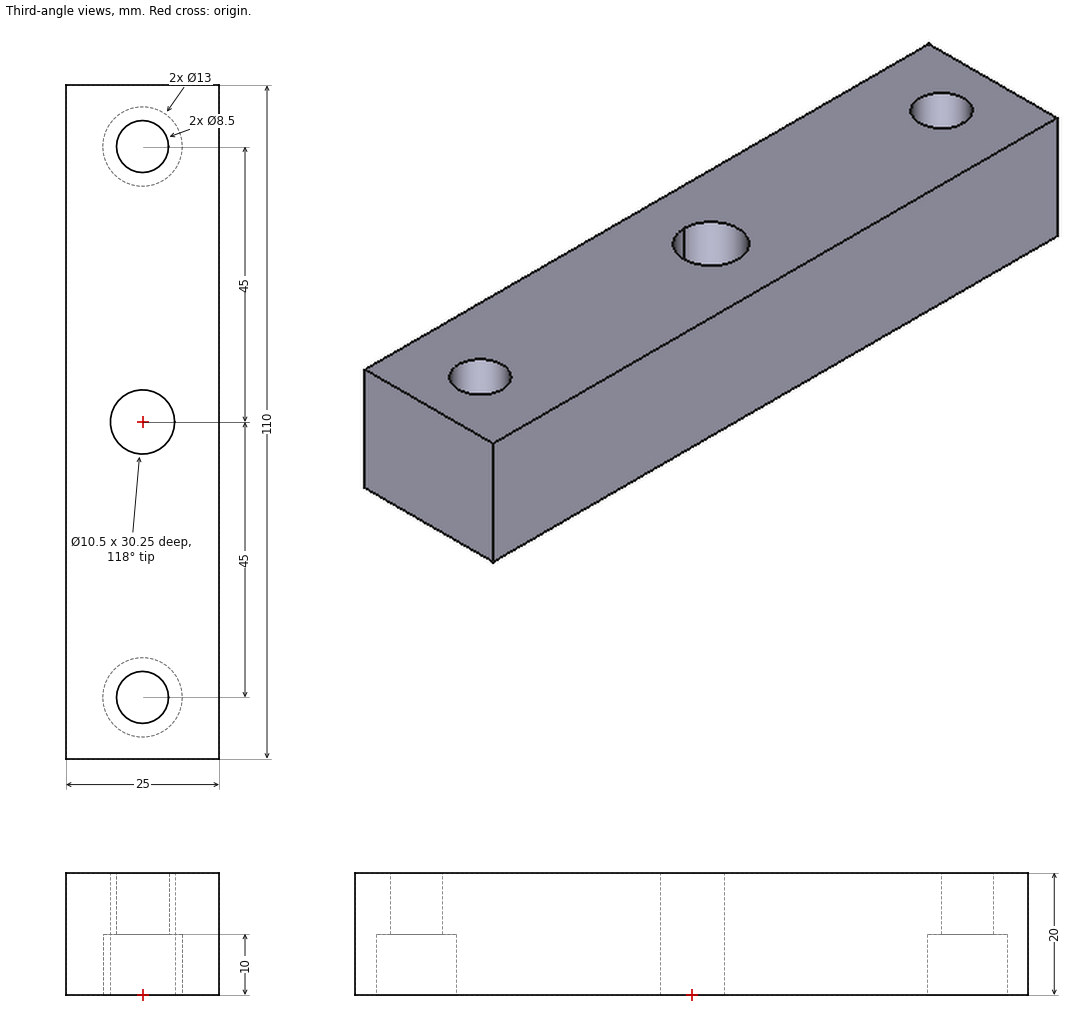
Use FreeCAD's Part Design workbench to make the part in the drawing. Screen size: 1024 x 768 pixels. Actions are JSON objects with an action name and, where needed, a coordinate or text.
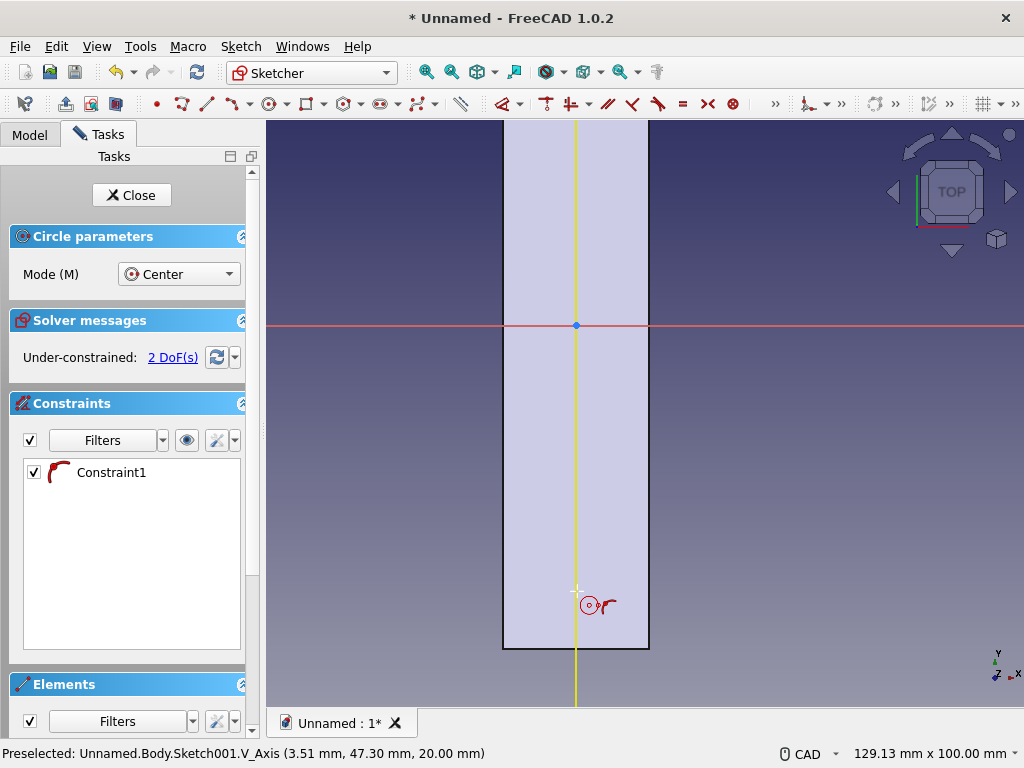
{"action": "left_click", "coordinate": [576, 590]}
{"action": "left_click", "coordinate": [594, 572]}
{"action": "key", "text": "Escape"}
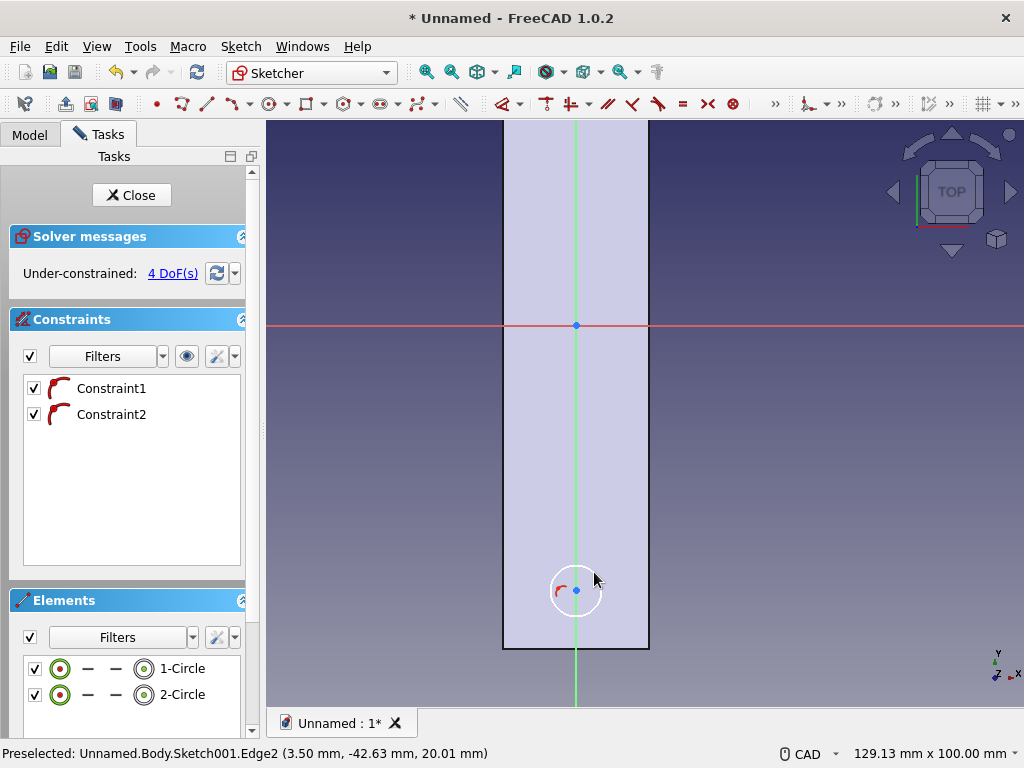
{"action": "scroll", "coordinate": [577, 592], "scroll_direction": "down", "scroll_amount": 2}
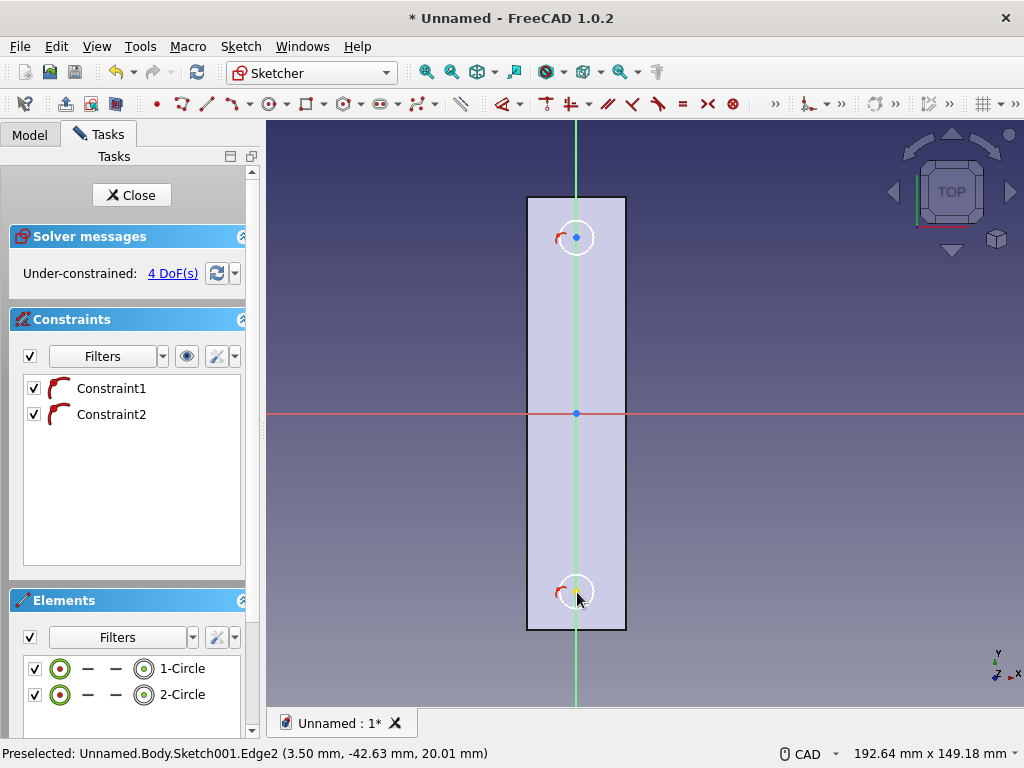
{"action": "left_click", "coordinate": [589, 226]}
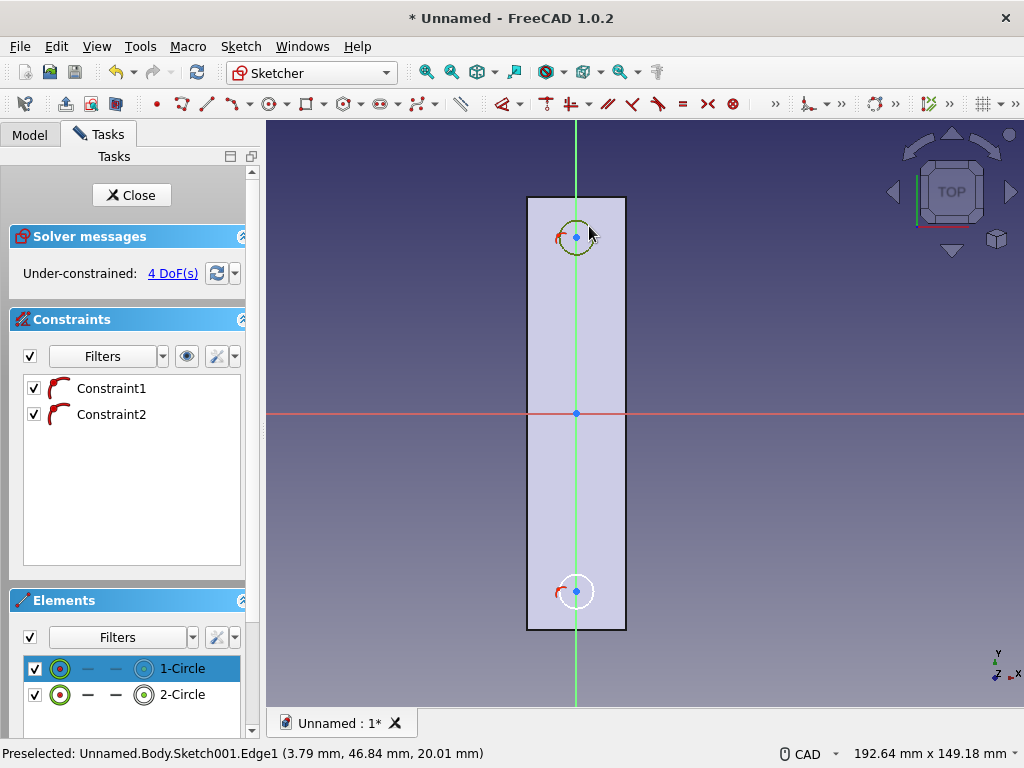
{"action": "left_click", "coordinate": [589, 580]}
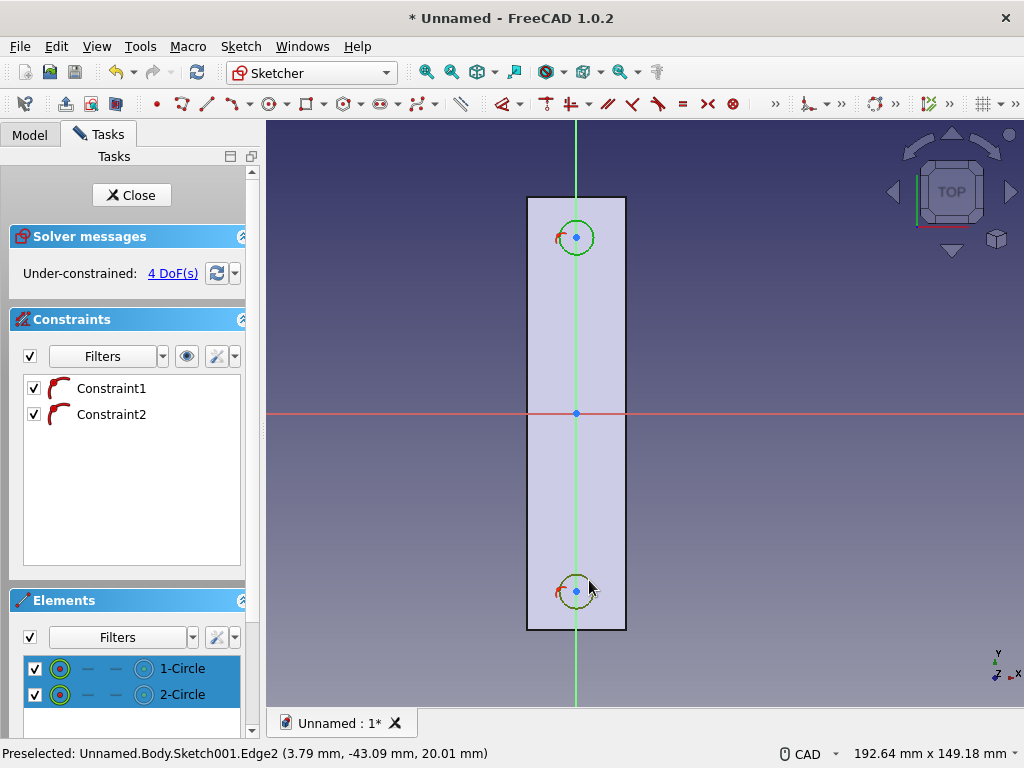
{"action": "left_click", "coordinate": [683, 104]}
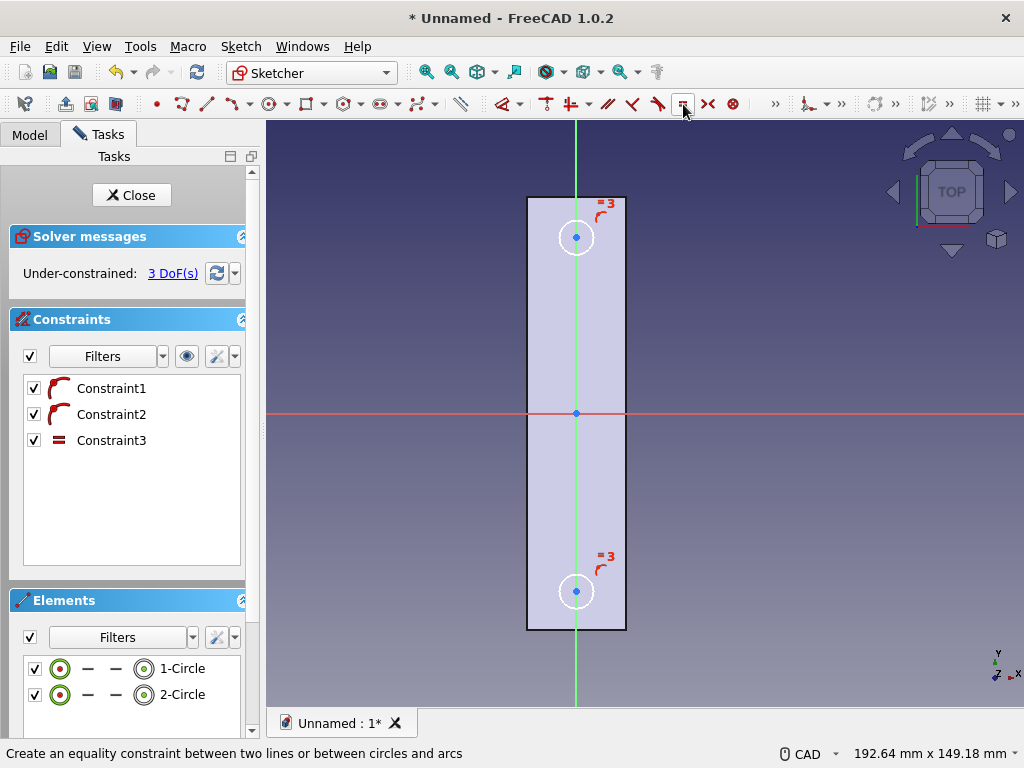
{"action": "left_click", "coordinate": [502, 104]}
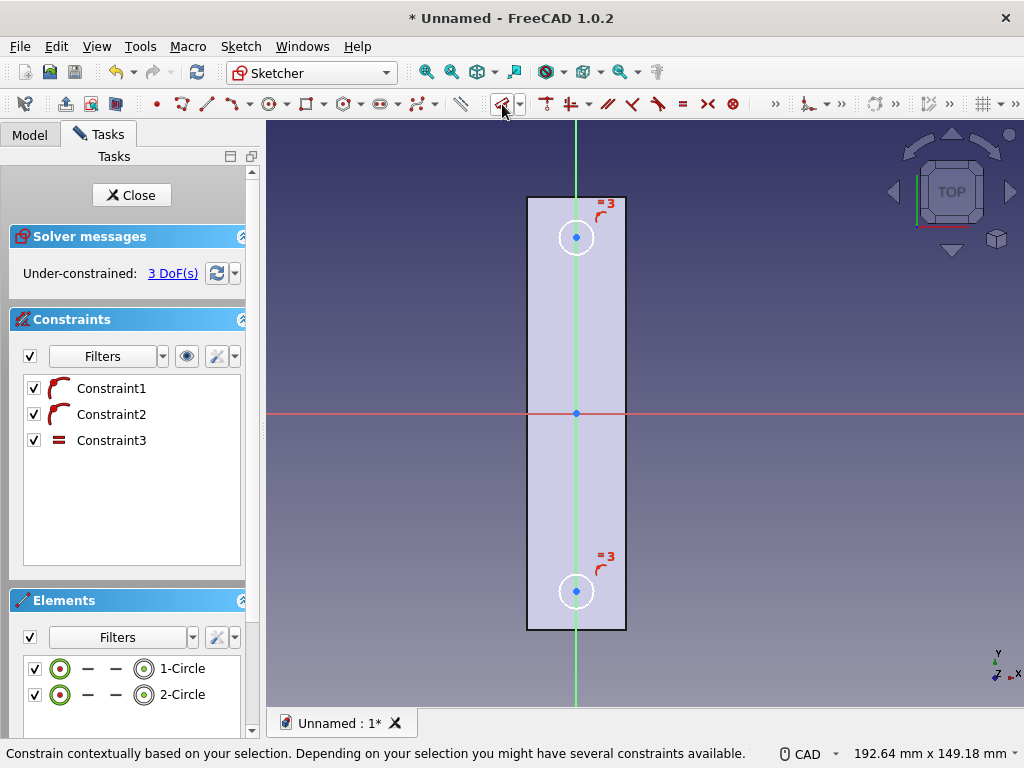
{"action": "left_click", "coordinate": [589, 226]}
{"action": "left_click", "coordinate": [612, 204]}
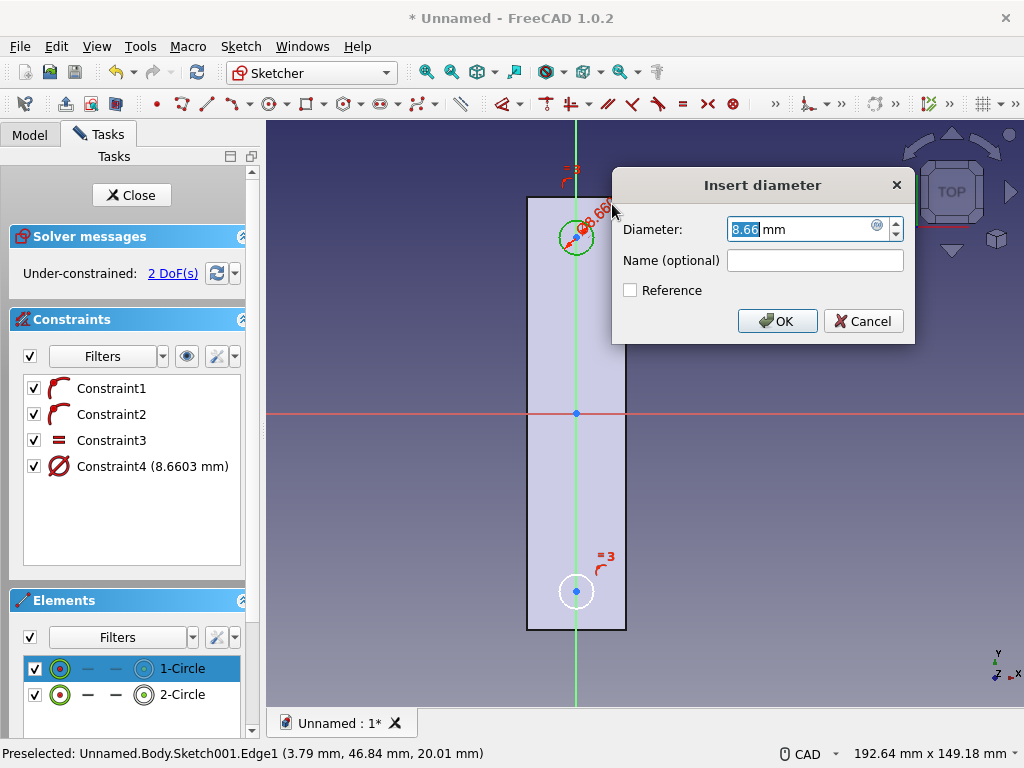
{"action": "type", "text": "8.5"}
{"action": "key", "text": "Return"}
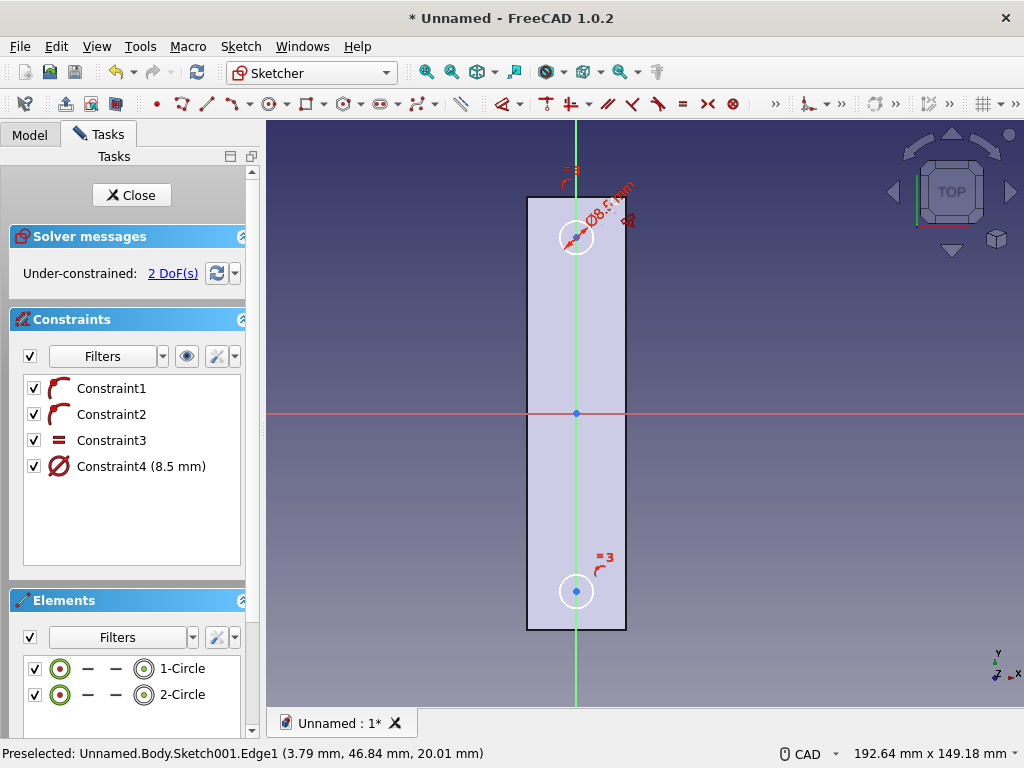
{"action": "left_click", "coordinate": [577, 238]}
{"action": "left_click", "coordinate": [611, 326]}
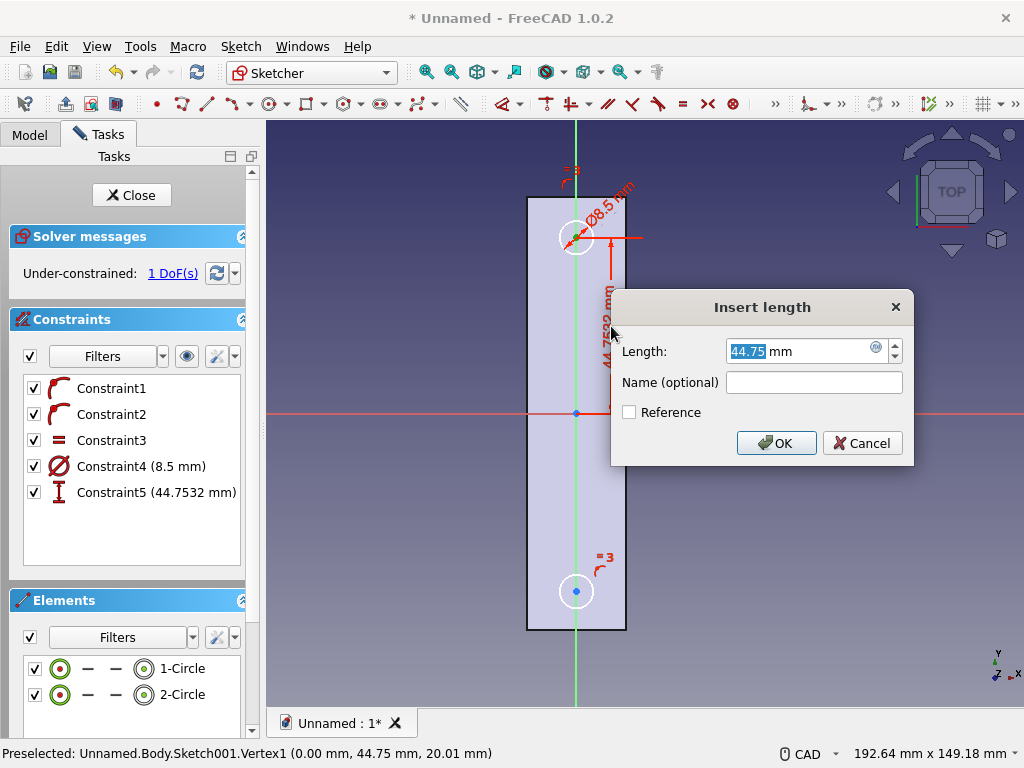
{"action": "type", "text": "45"}
{"action": "key", "text": "Return"}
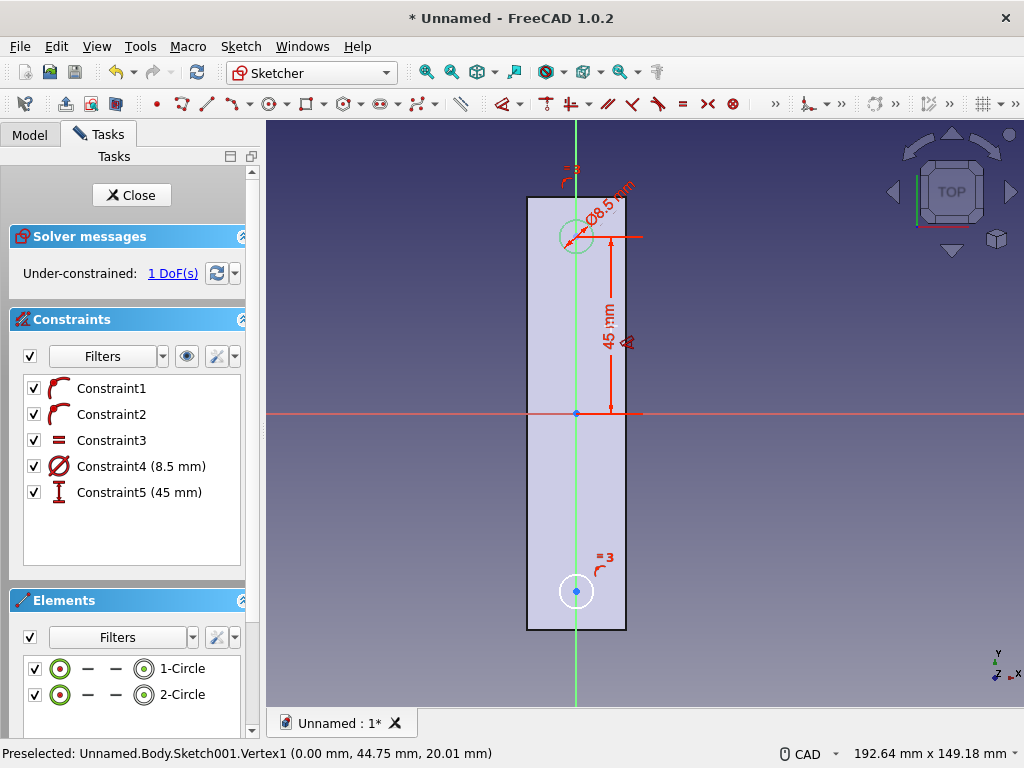
{"action": "left_click", "coordinate": [577, 592]}
{"action": "left_click", "coordinate": [611, 503]}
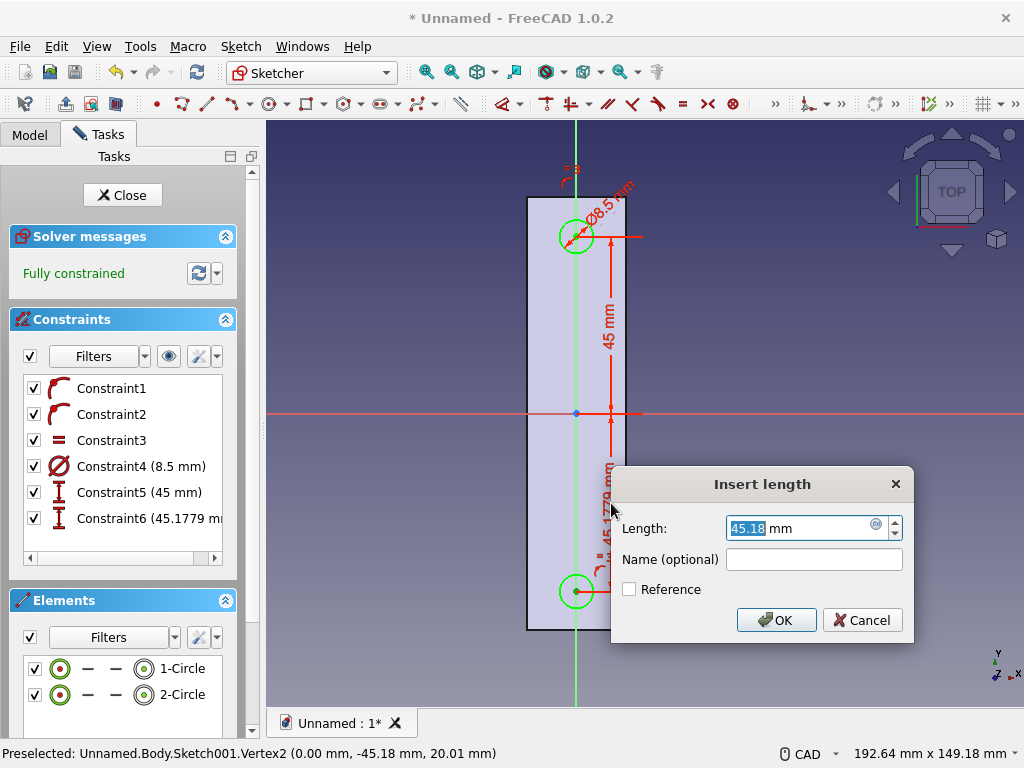
{"action": "type", "text": "45"}
{"action": "key", "text": "Return"}
{"action": "key", "text": "Escape"}